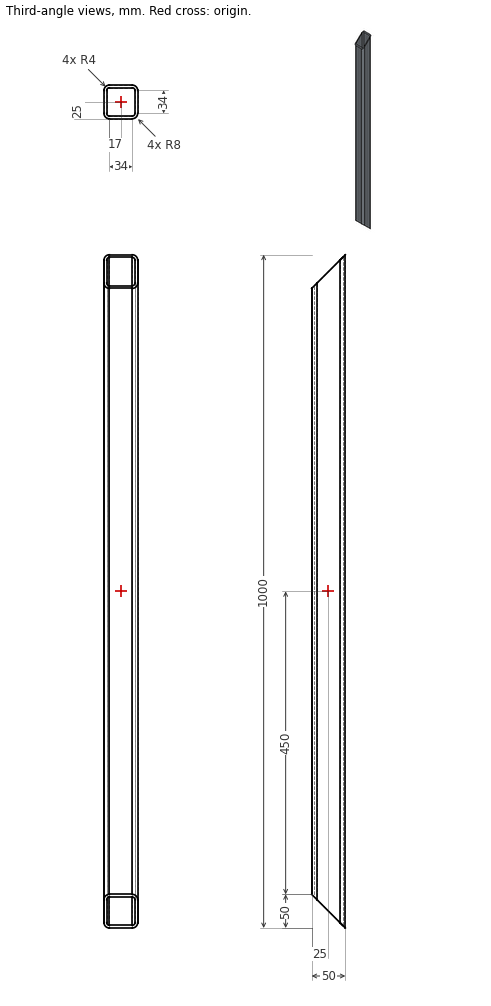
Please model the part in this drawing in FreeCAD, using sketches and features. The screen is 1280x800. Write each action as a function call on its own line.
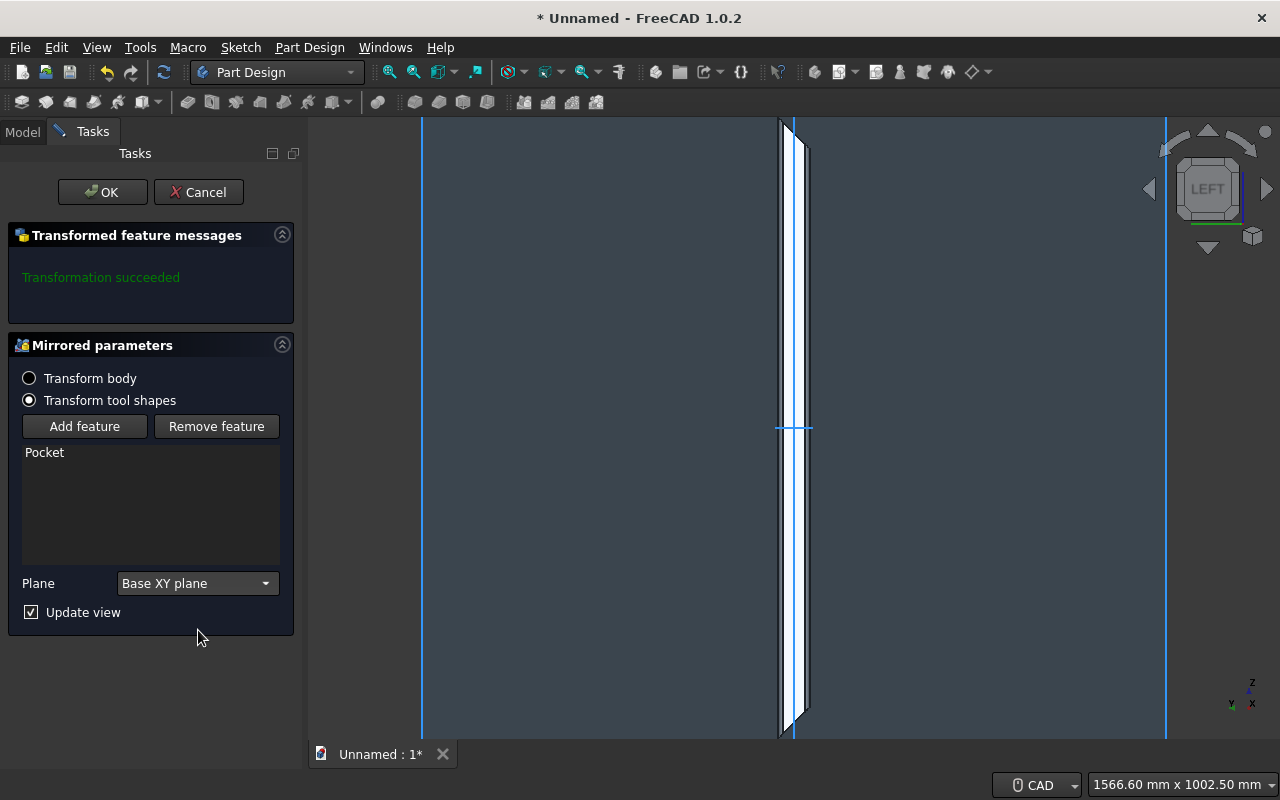
click(103, 192)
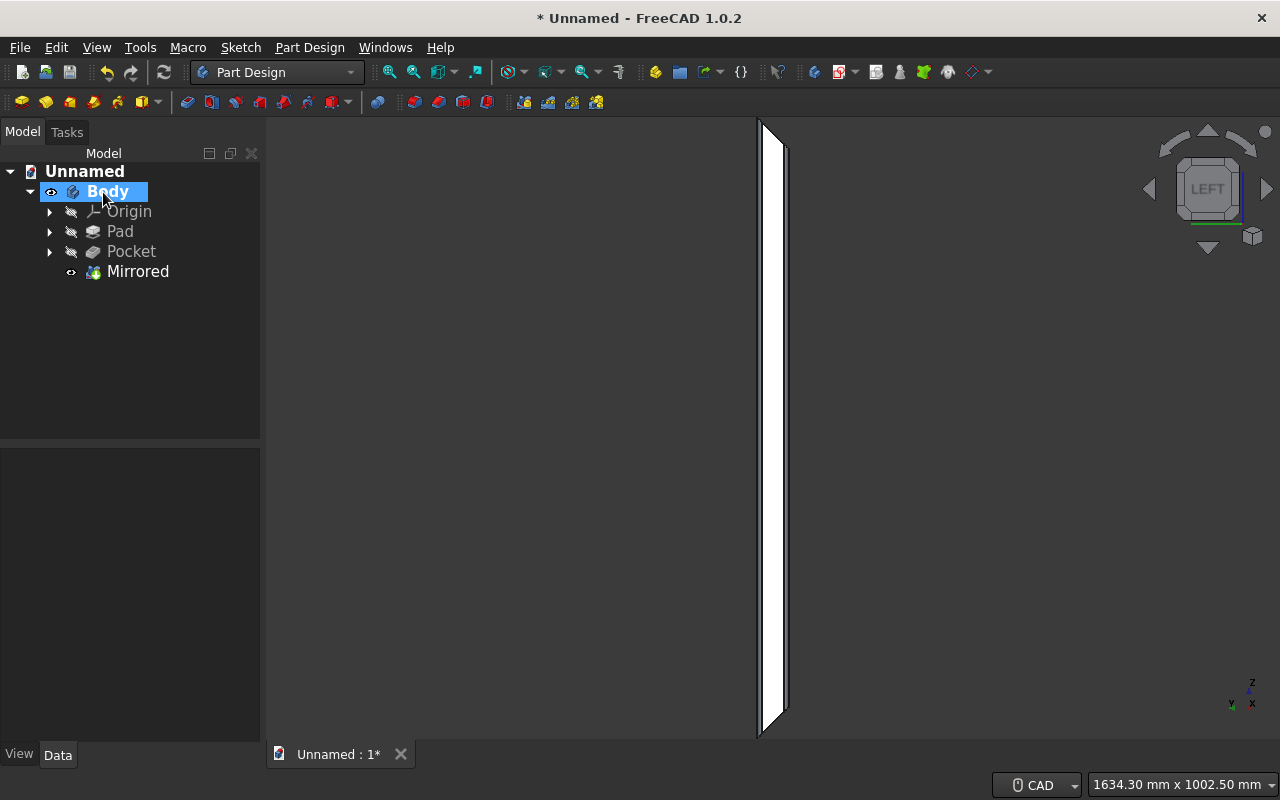
key(0)